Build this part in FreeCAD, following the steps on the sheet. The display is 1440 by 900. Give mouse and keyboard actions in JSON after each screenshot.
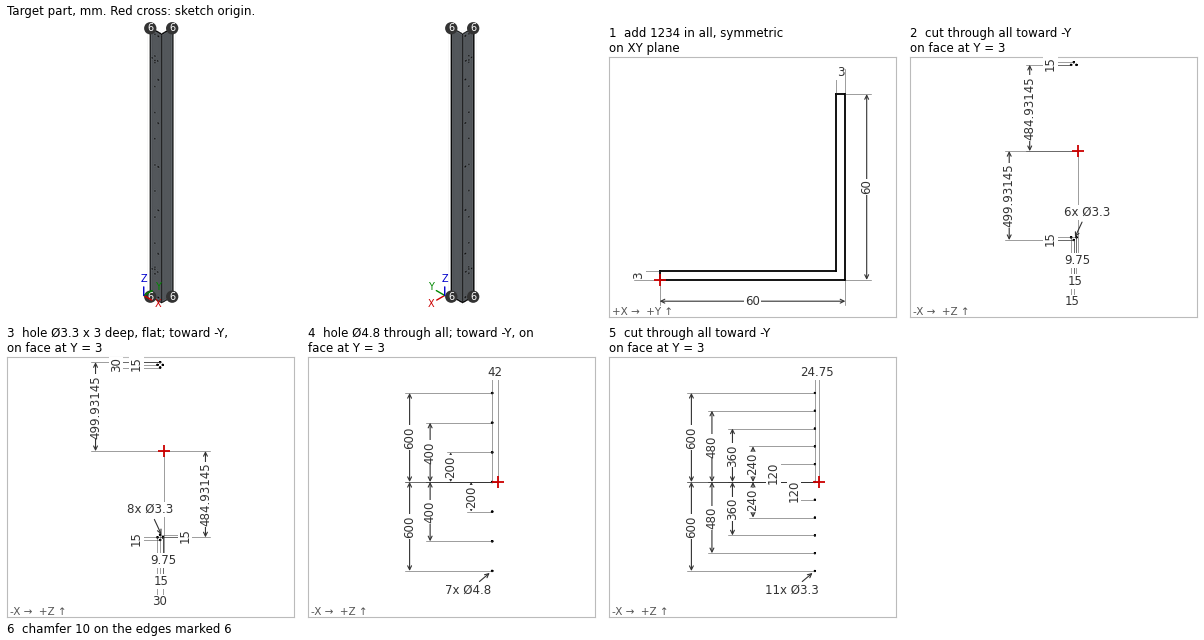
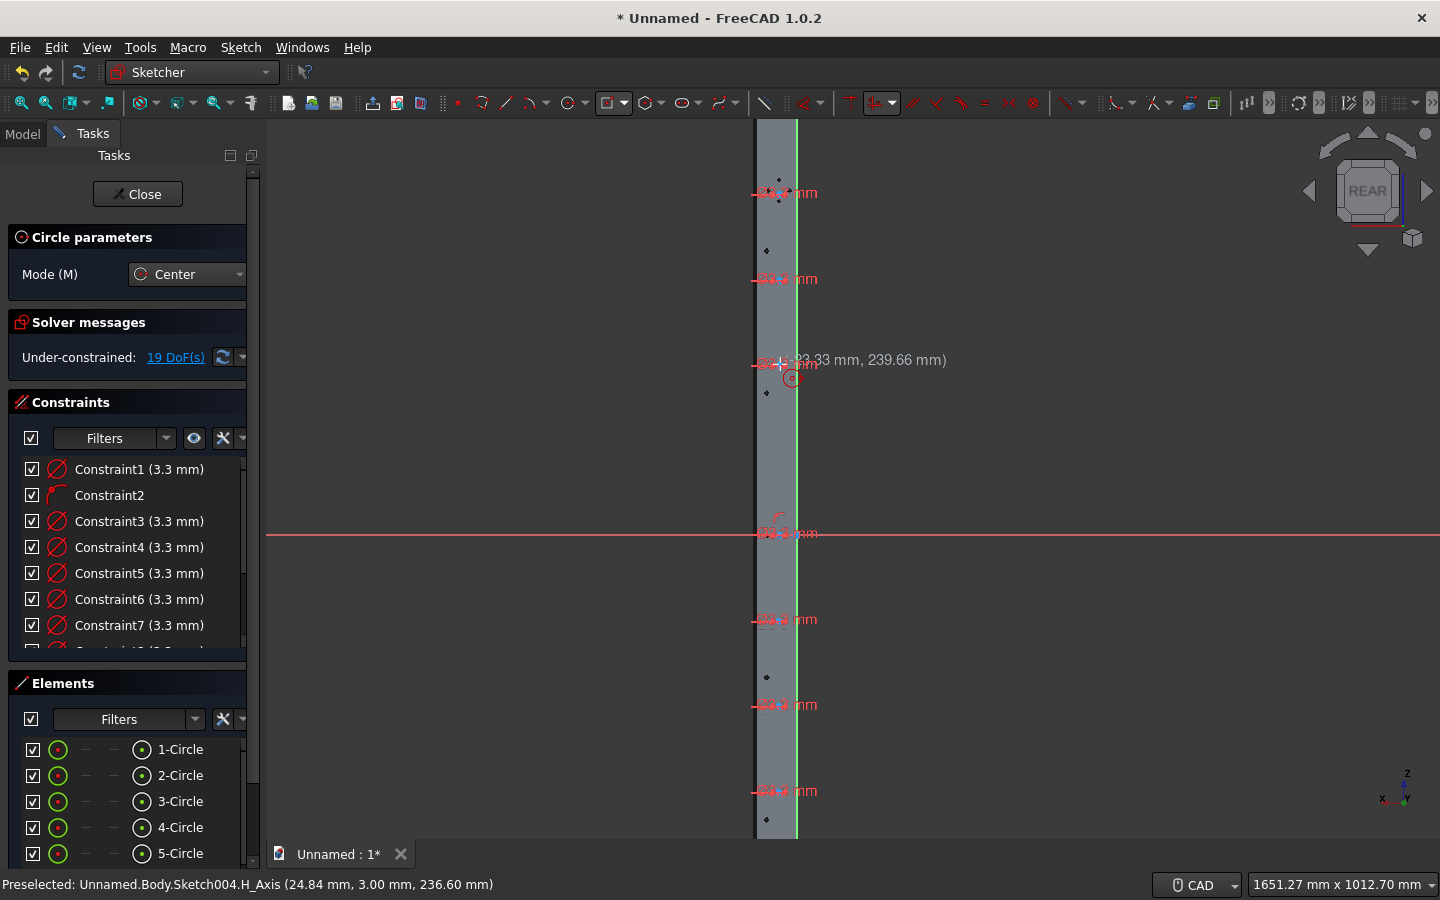
{"action": "scroll", "coordinate": [779, 450], "scroll_direction": "up", "scroll_amount": 15}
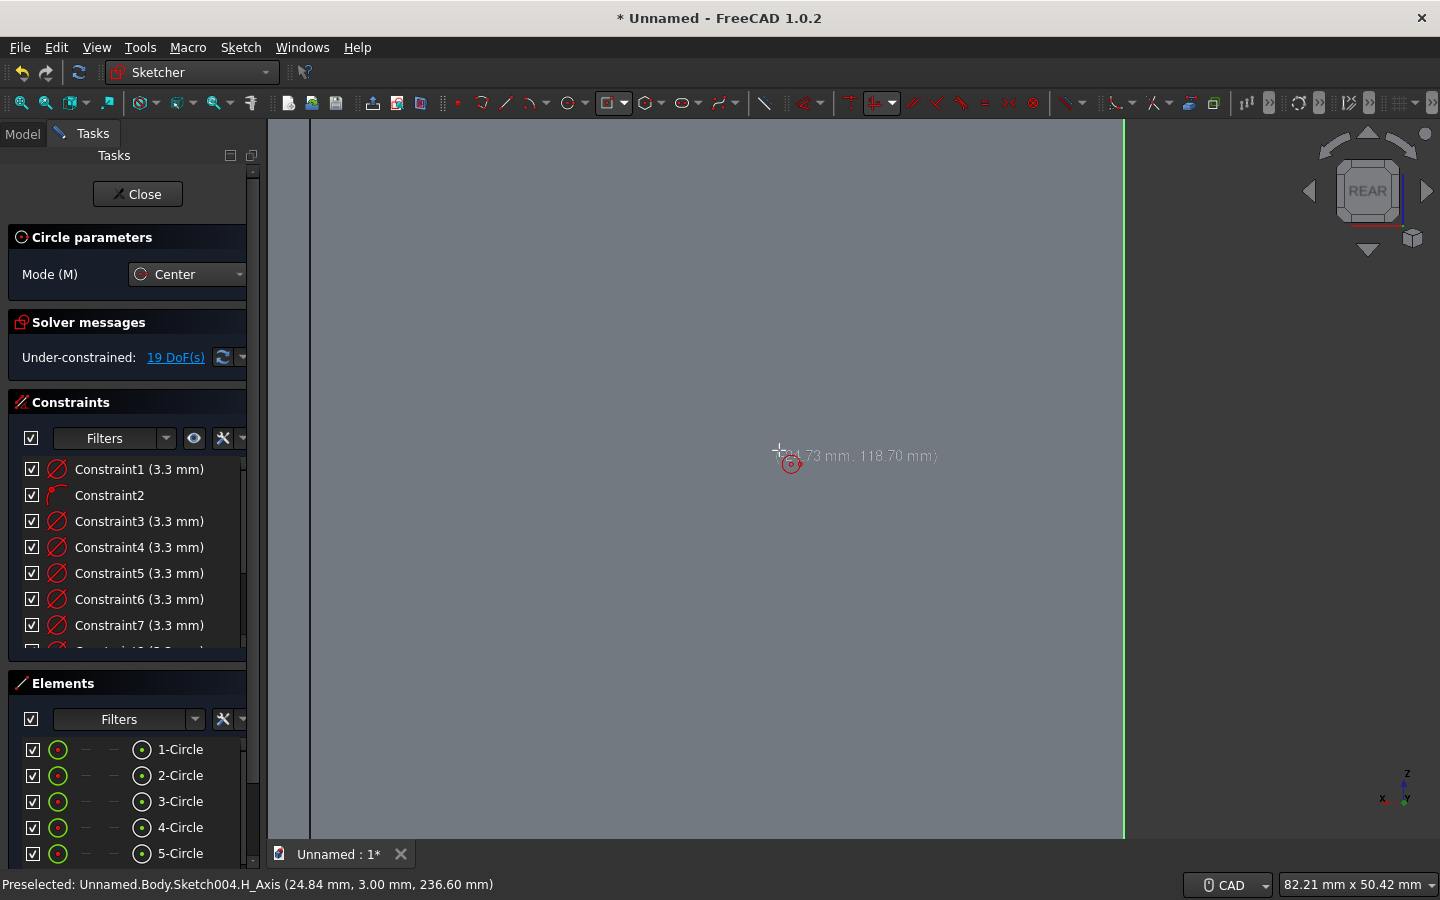
{"action": "scroll", "coordinate": [779, 421], "scroll_direction": "down", "scroll_amount": 17}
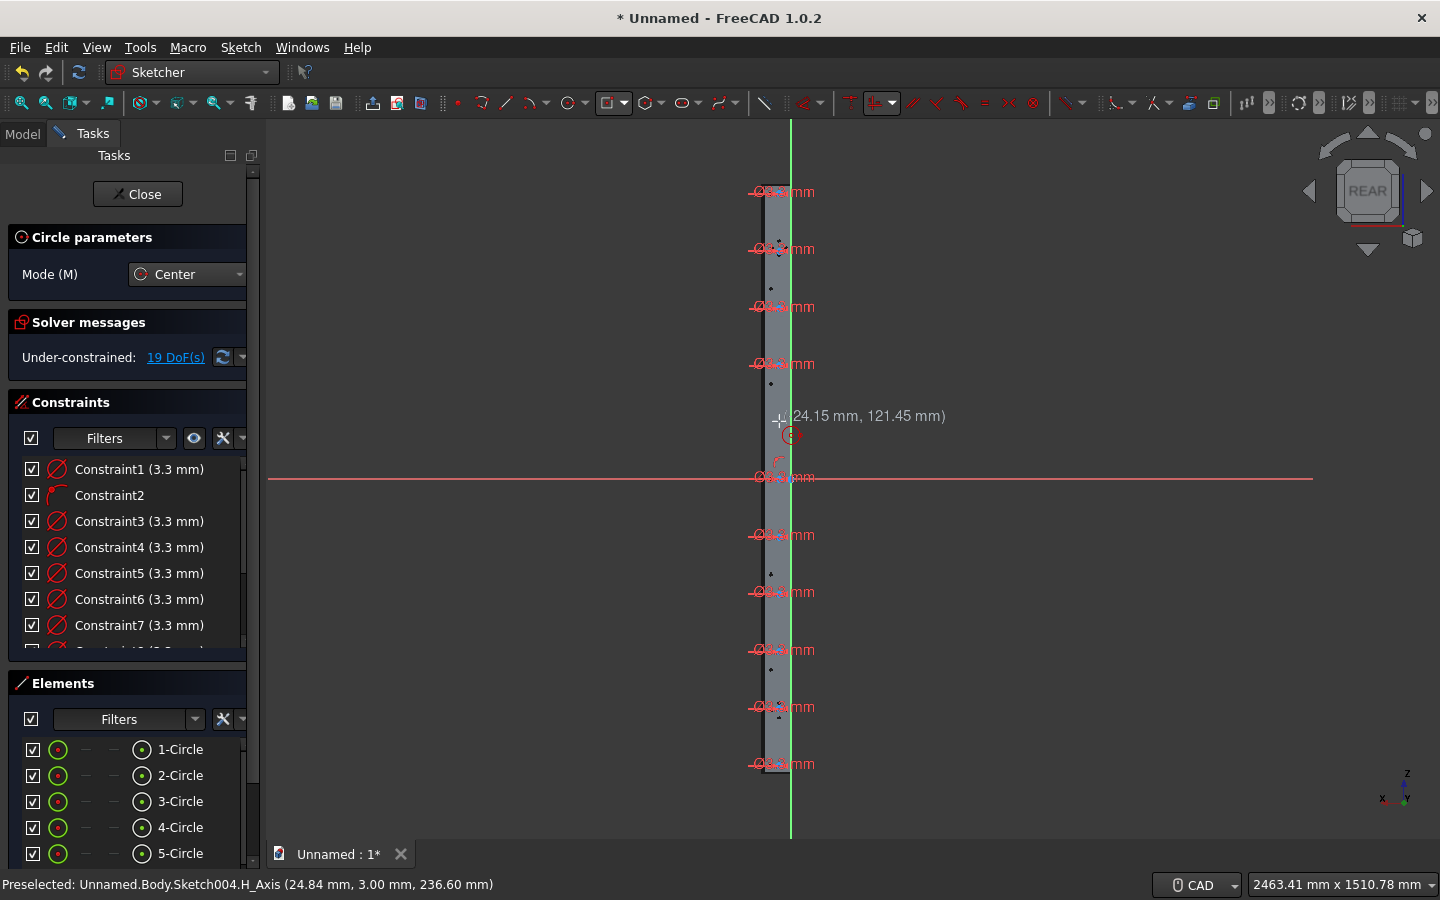
{"action": "scroll", "coordinate": [779, 422], "scroll_direction": "up", "scroll_amount": 2}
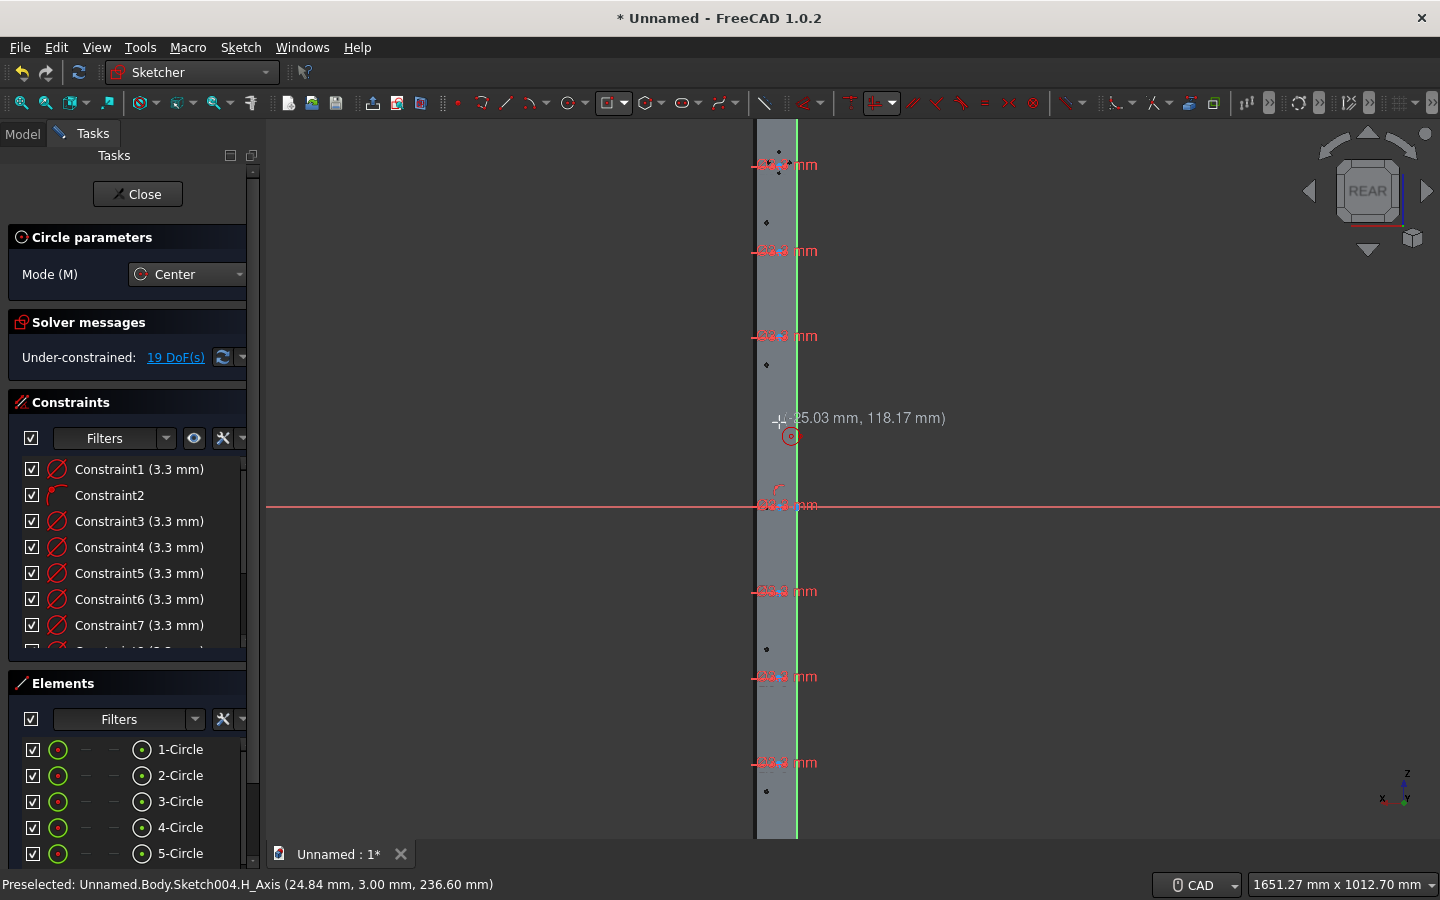
{"action": "left_click", "coordinate": [779, 422]}
{"action": "mouse_move", "coordinate": [780, 421]}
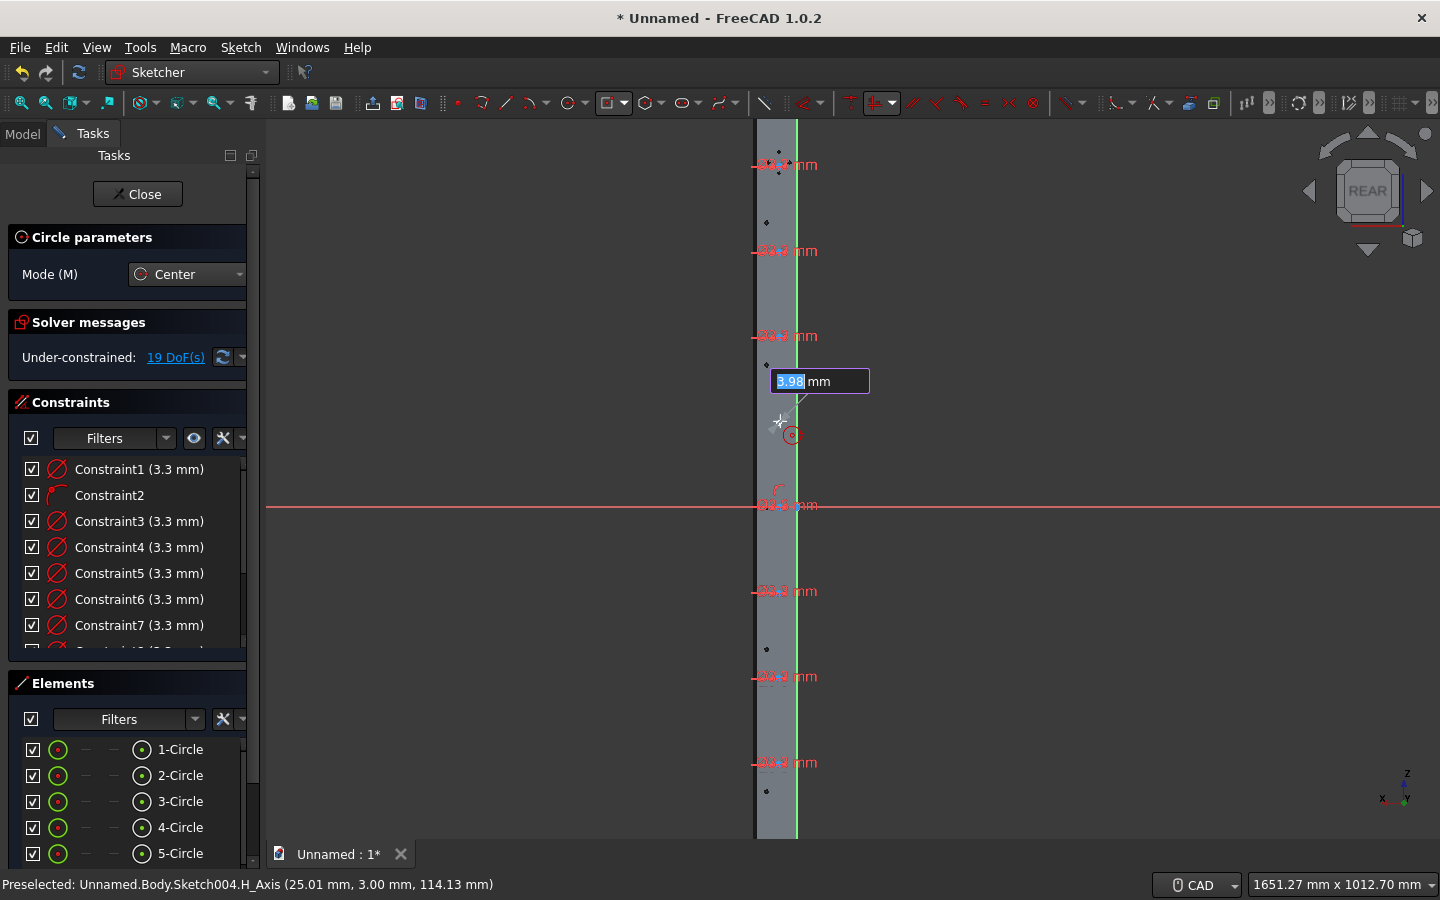
{"action": "type", "text": "3.3"}
{"action": "key", "text": "Return"}
{"action": "key", "text": "Escape"}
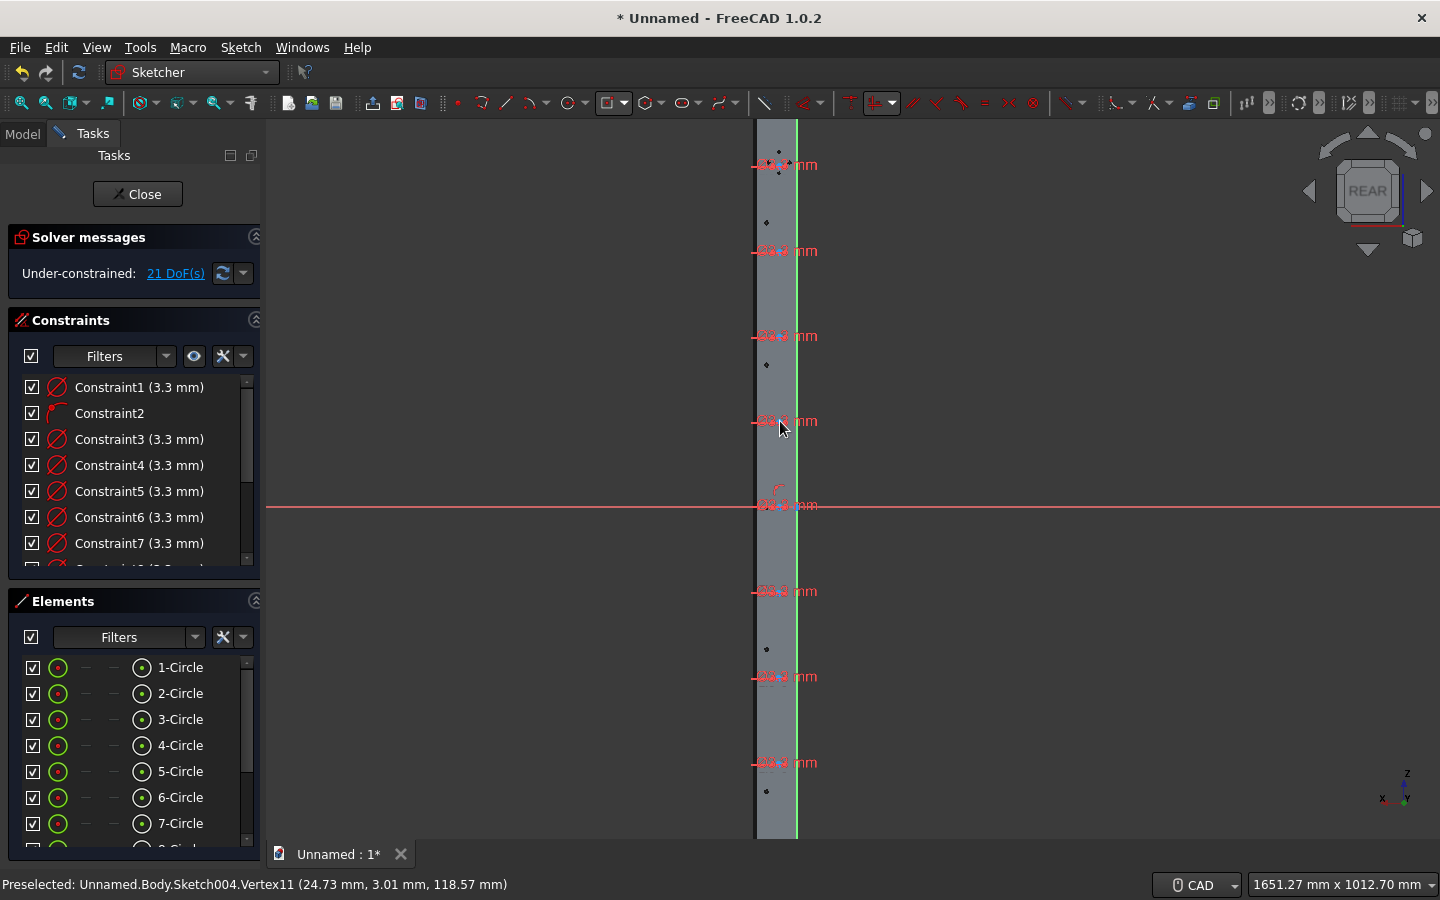
{"action": "left_click", "coordinate": [779, 507]}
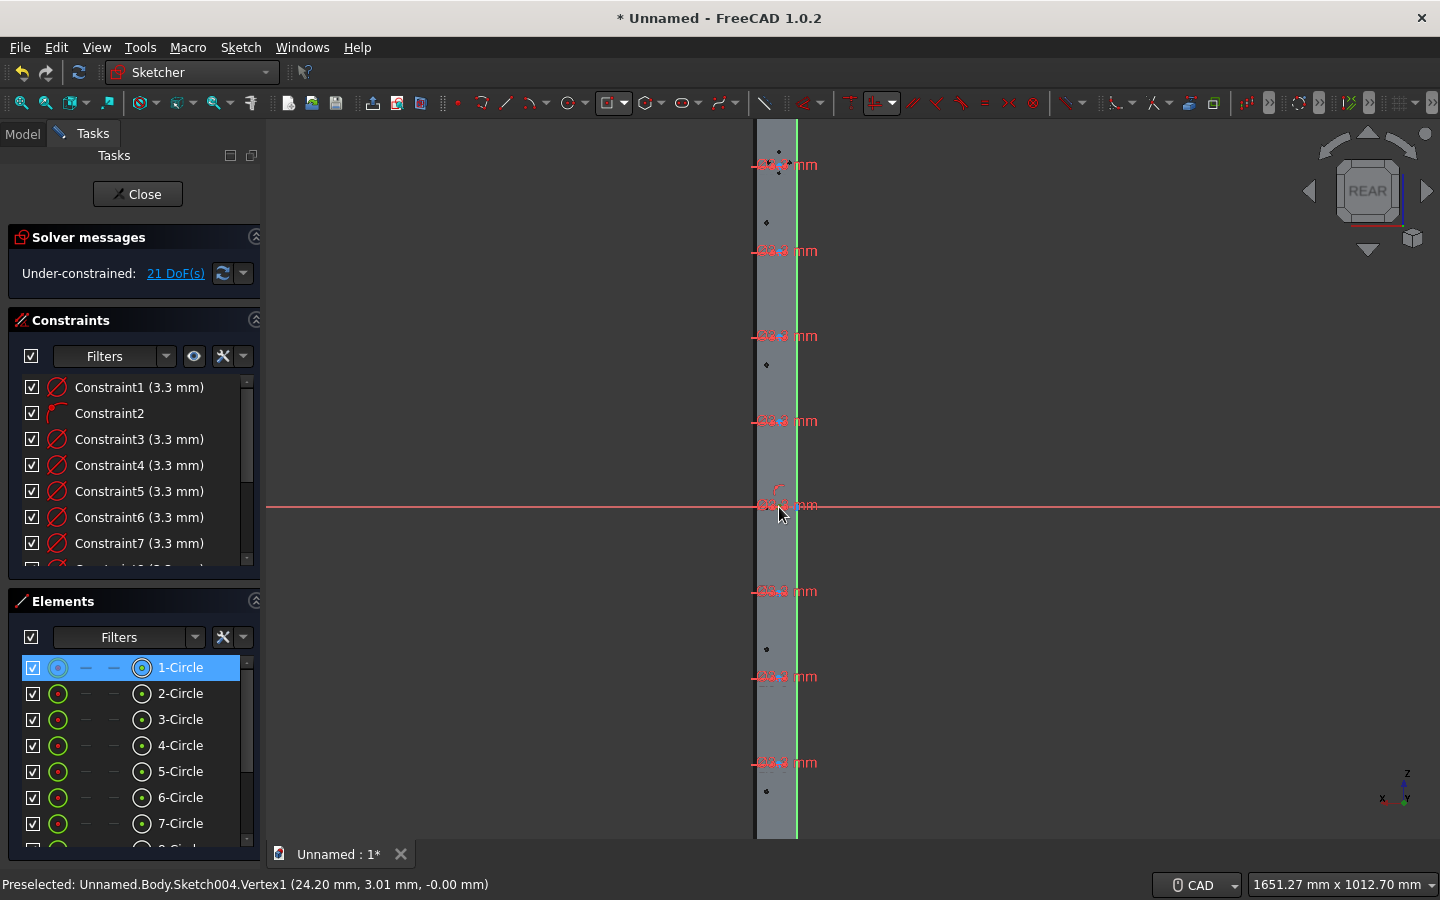
{"action": "left_click", "coordinate": [779, 593]}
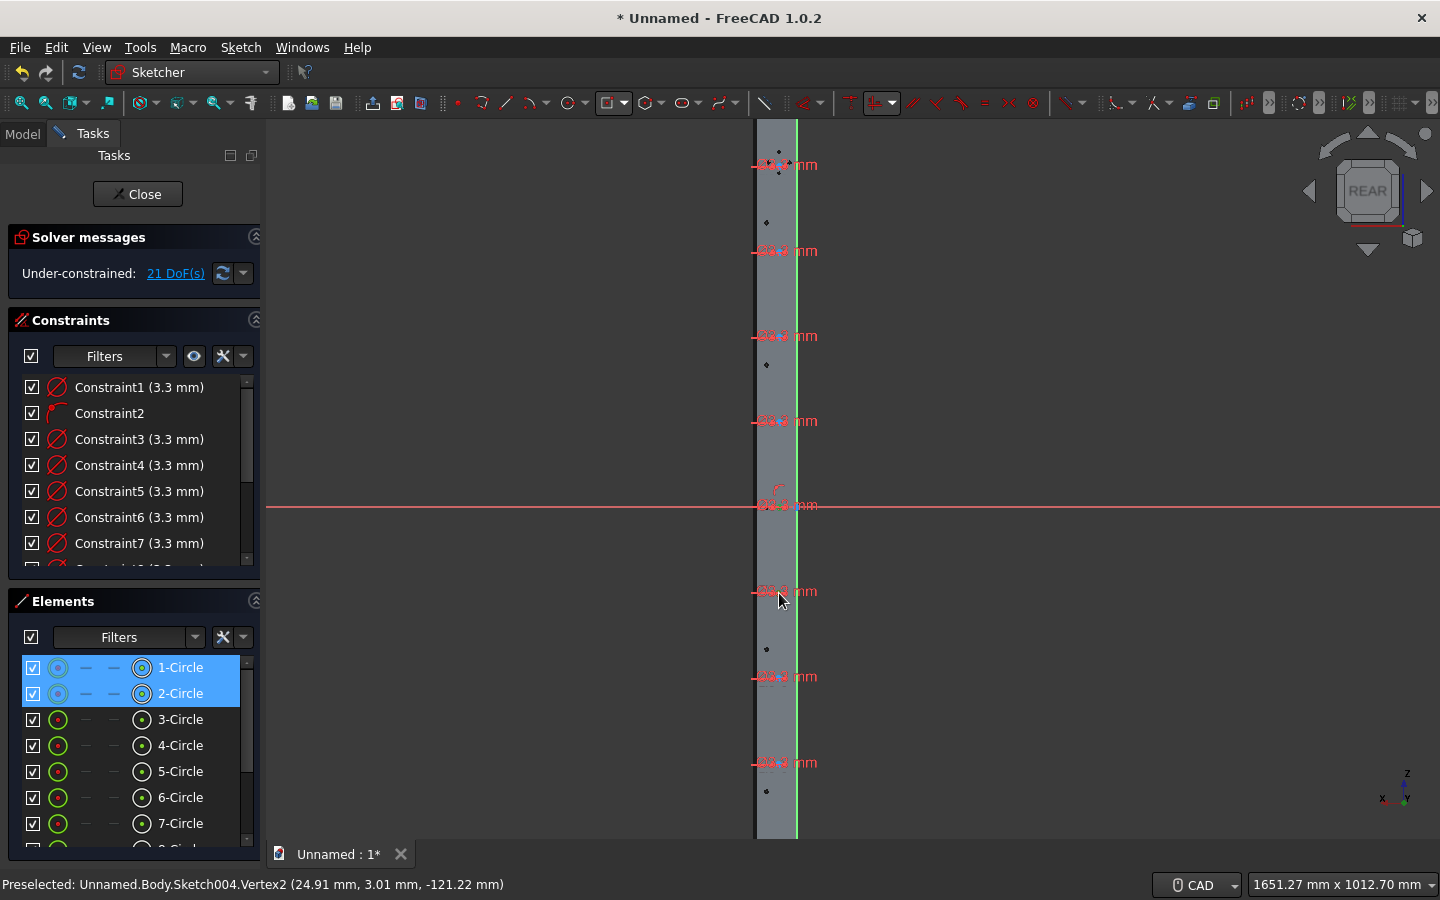
{"action": "key", "text": "v"}